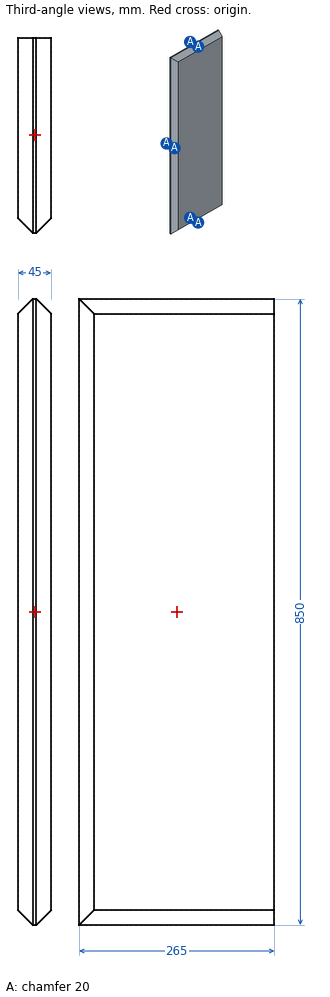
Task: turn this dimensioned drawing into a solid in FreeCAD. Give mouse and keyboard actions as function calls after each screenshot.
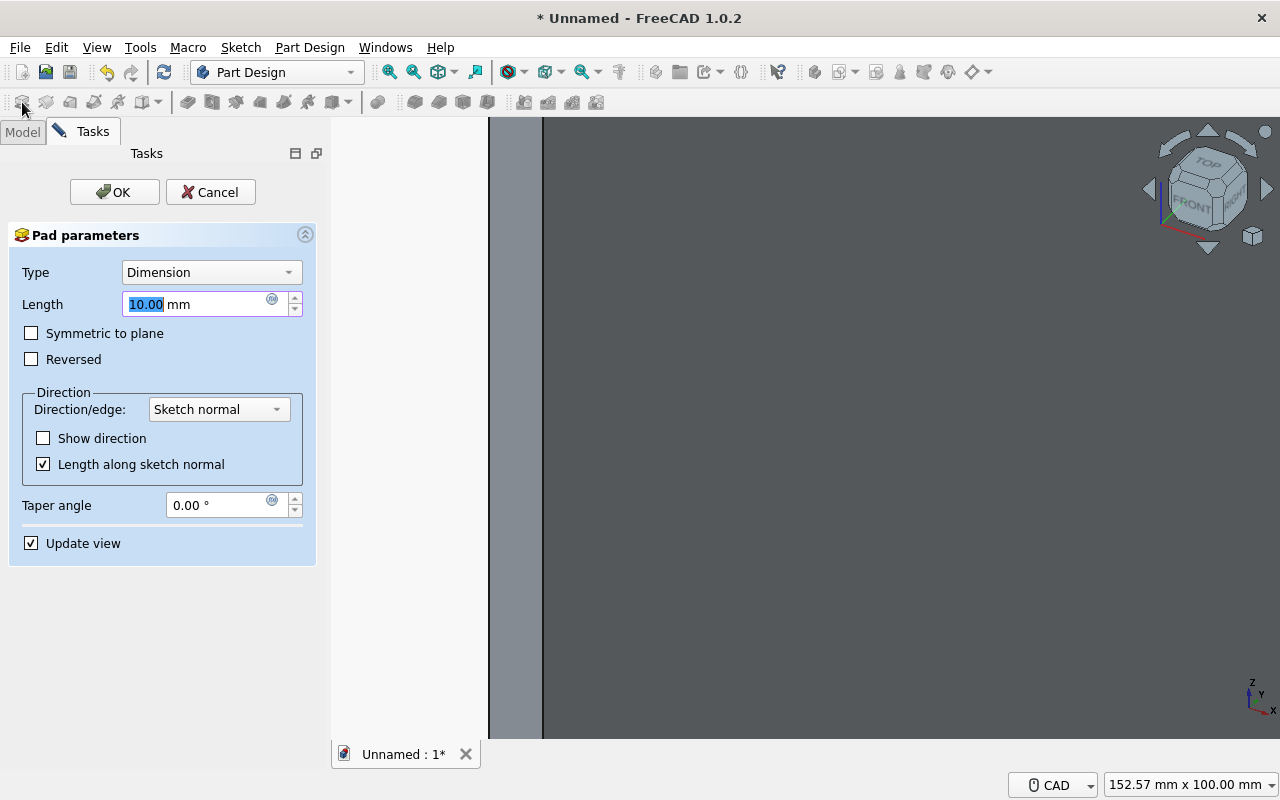
text(45)
key(Tab)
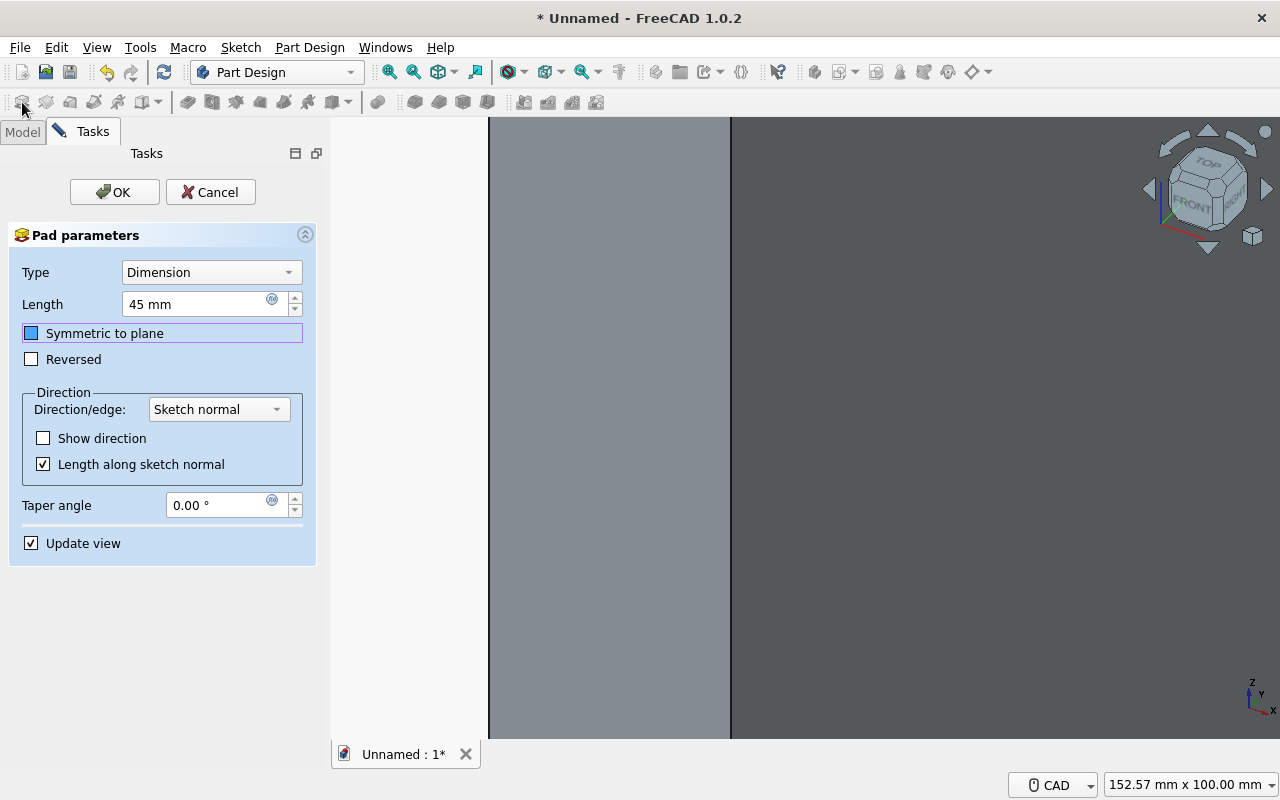
click(30, 333)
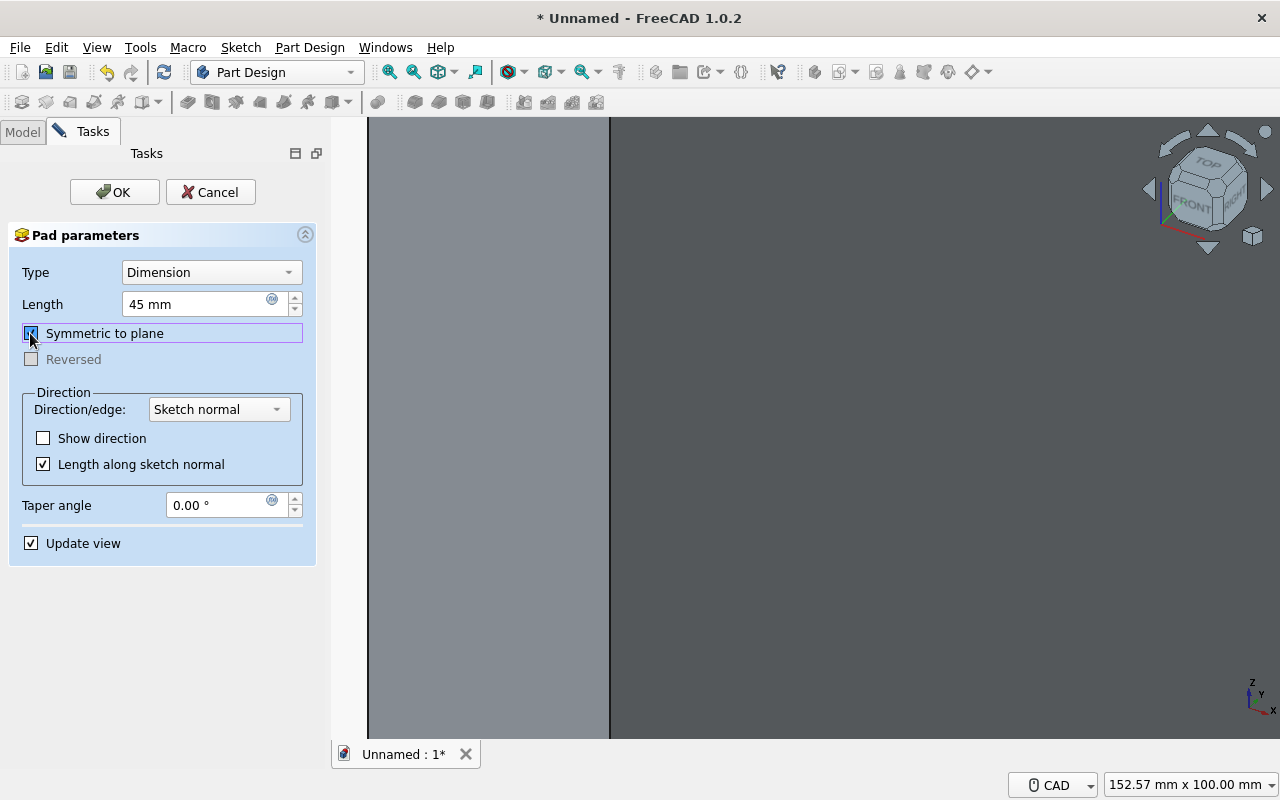
click(115, 192)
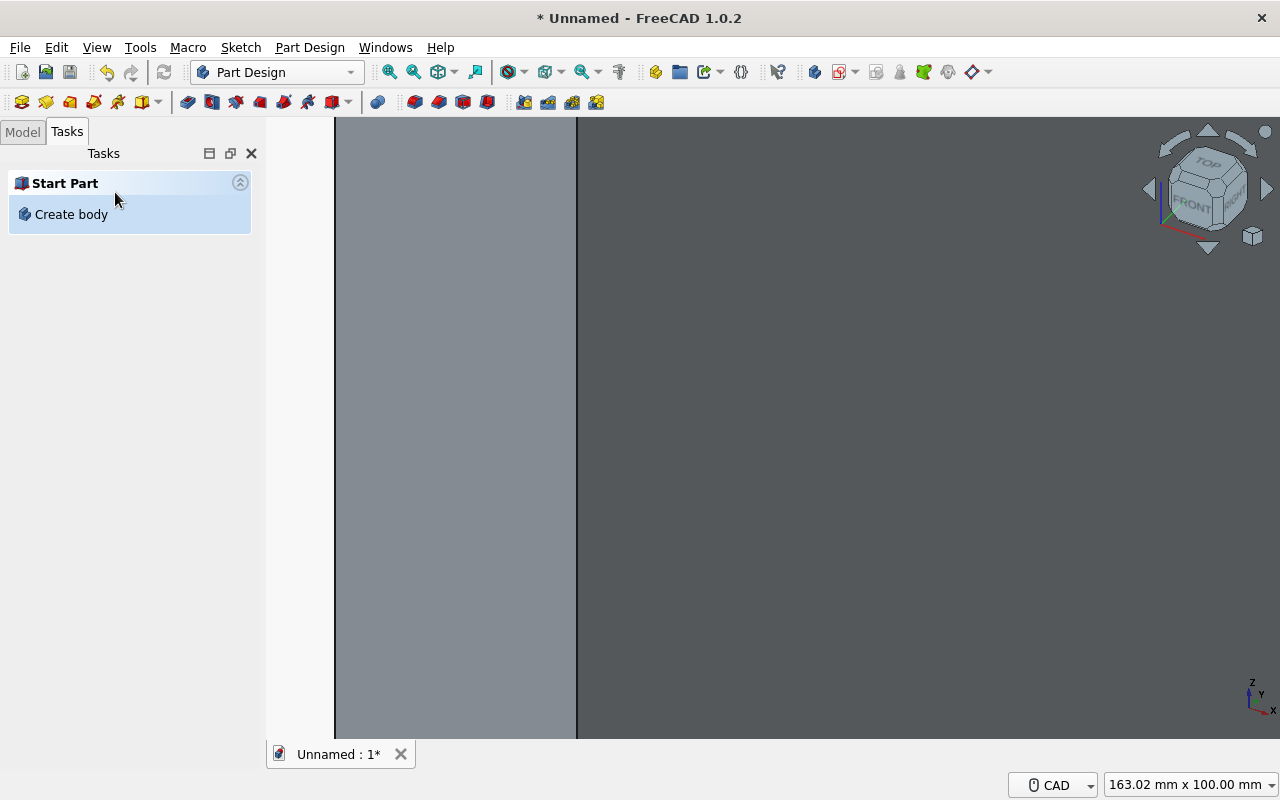
key(v)
key(f)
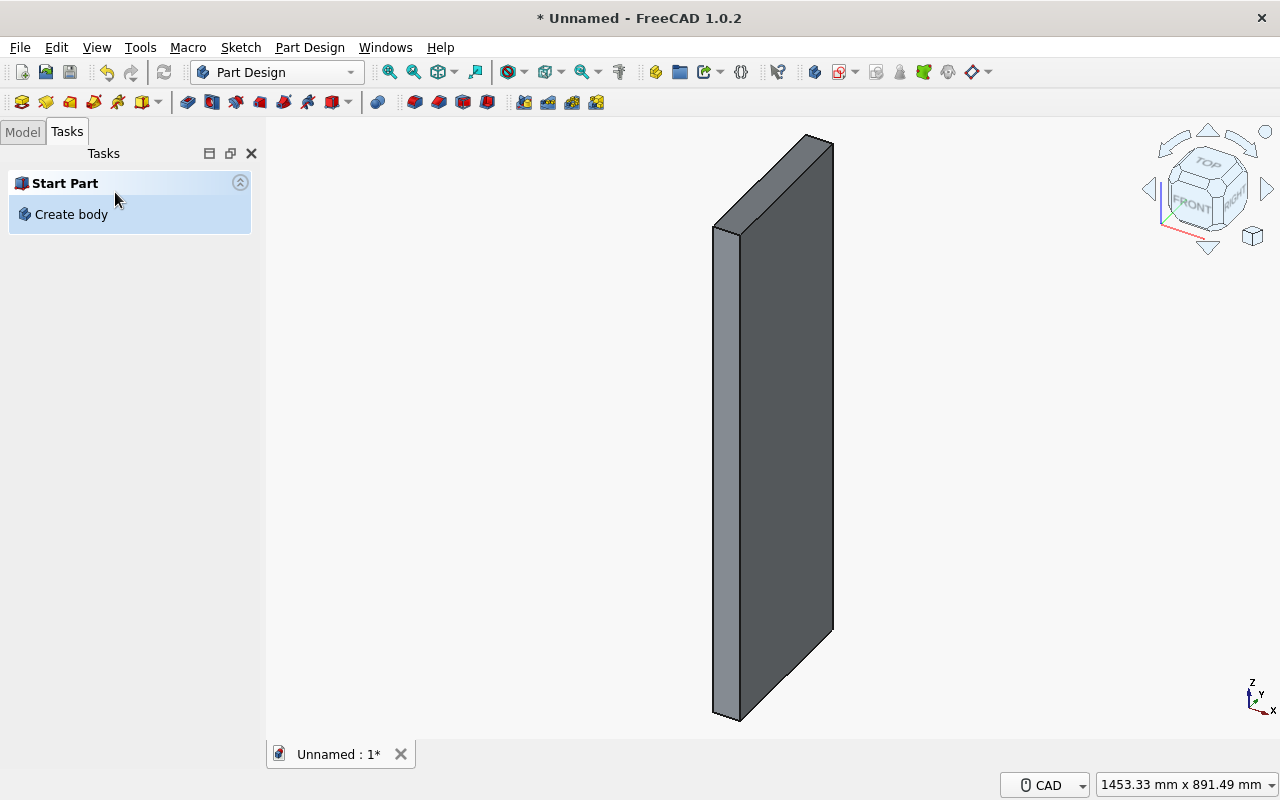
click(787, 189)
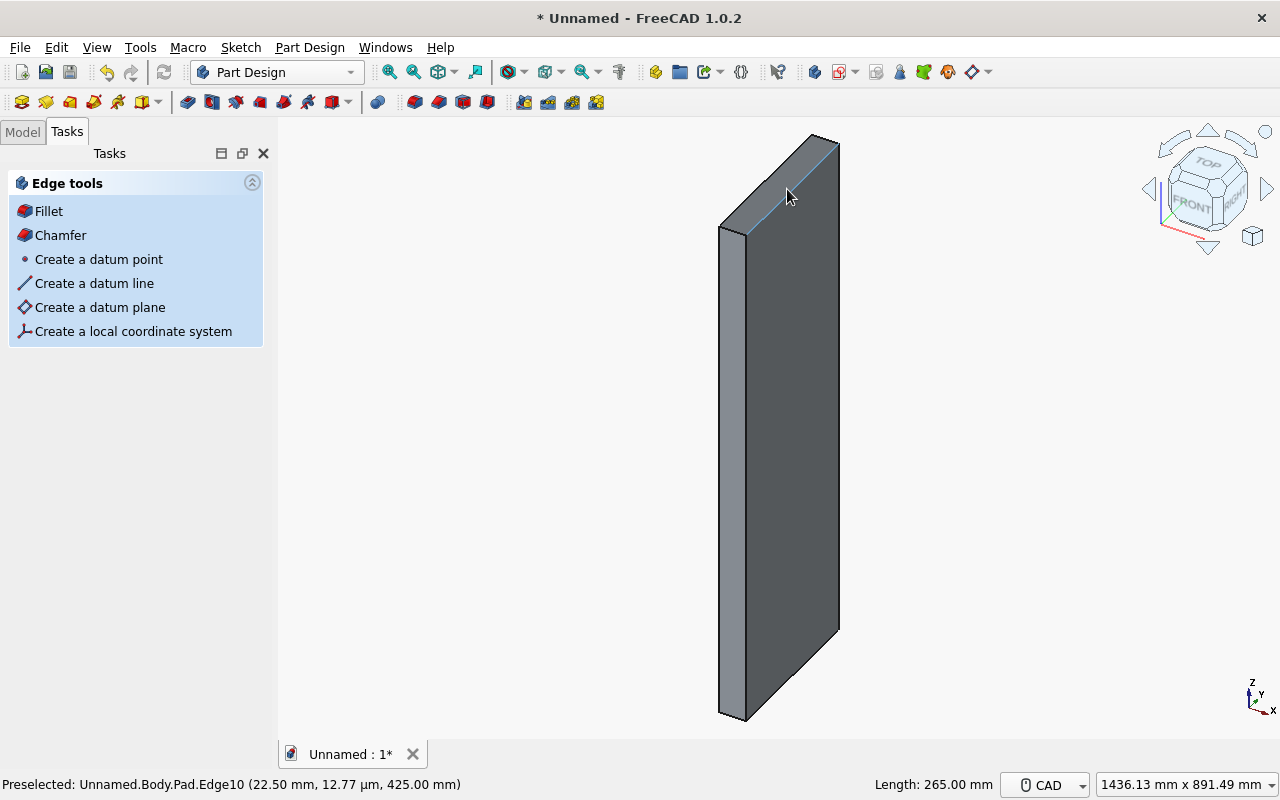
click(746, 477, ctrl)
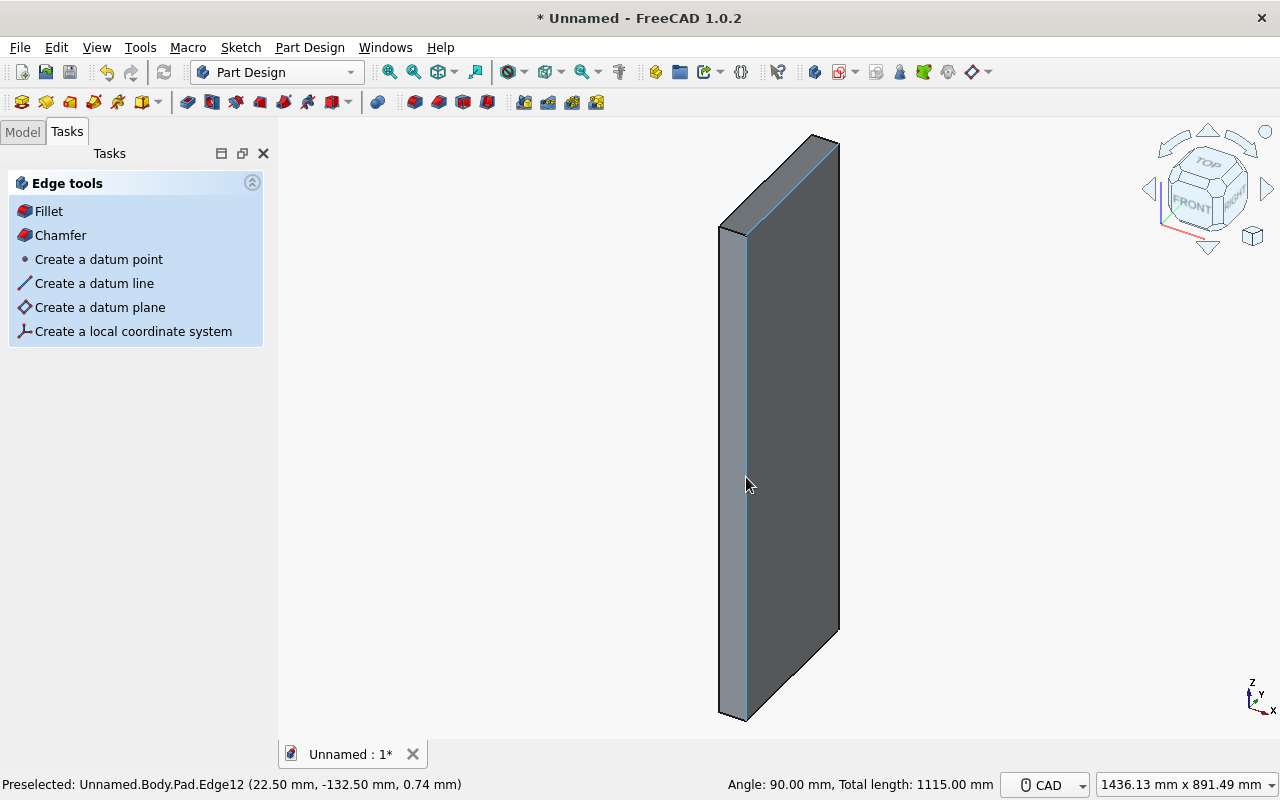
key(0)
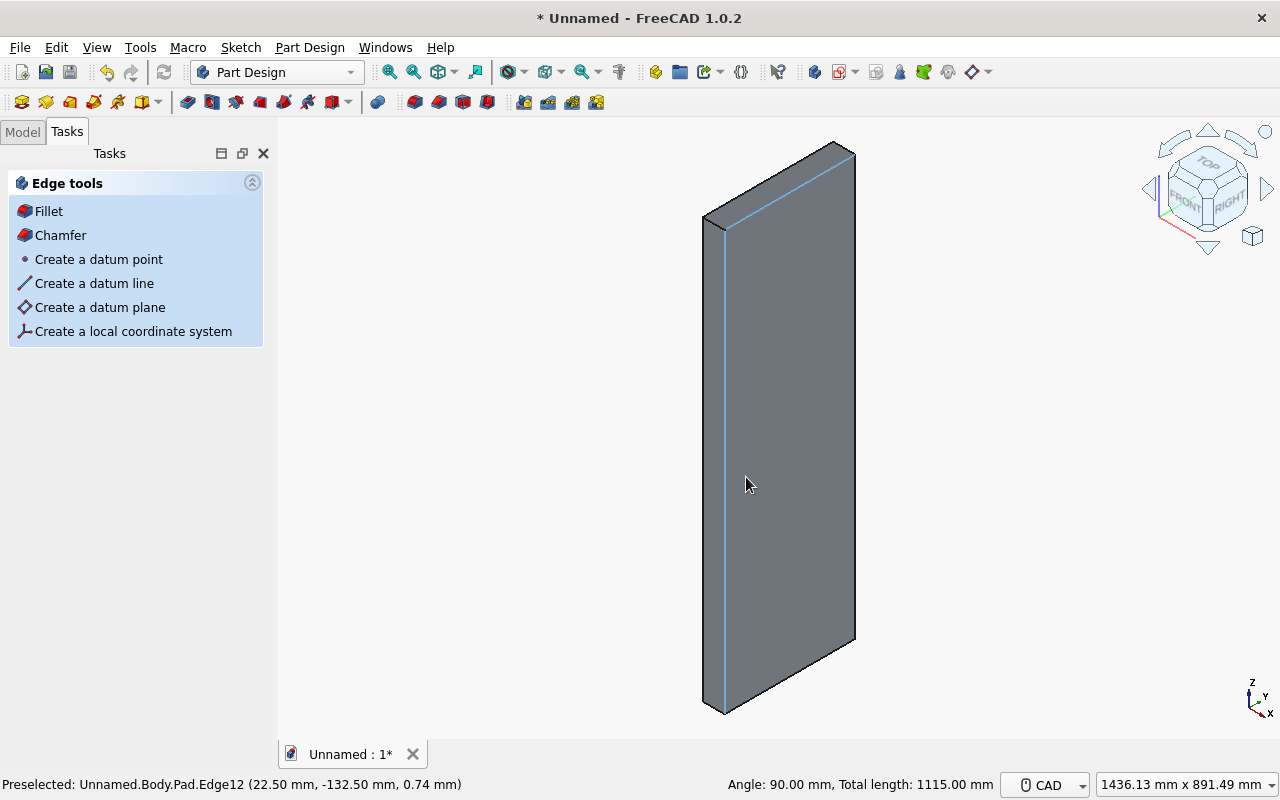
key(2)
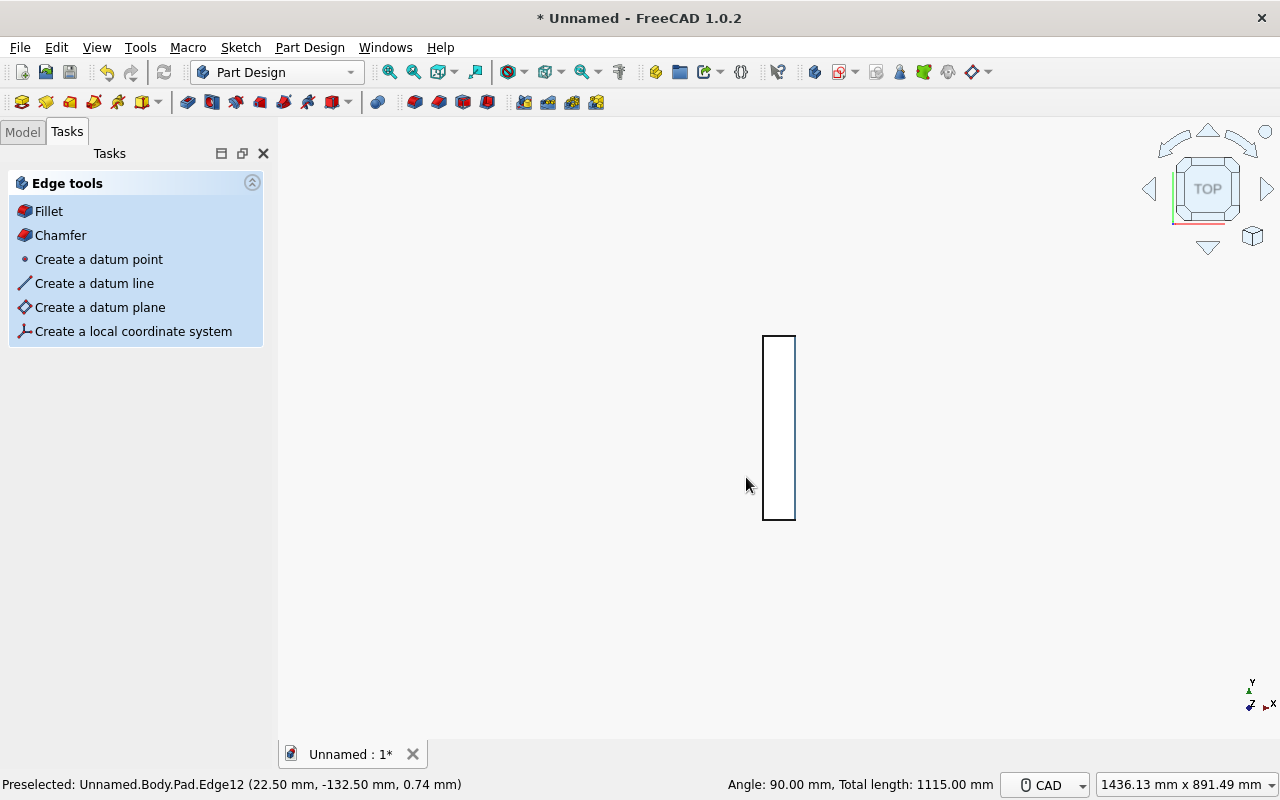
click(390, 72)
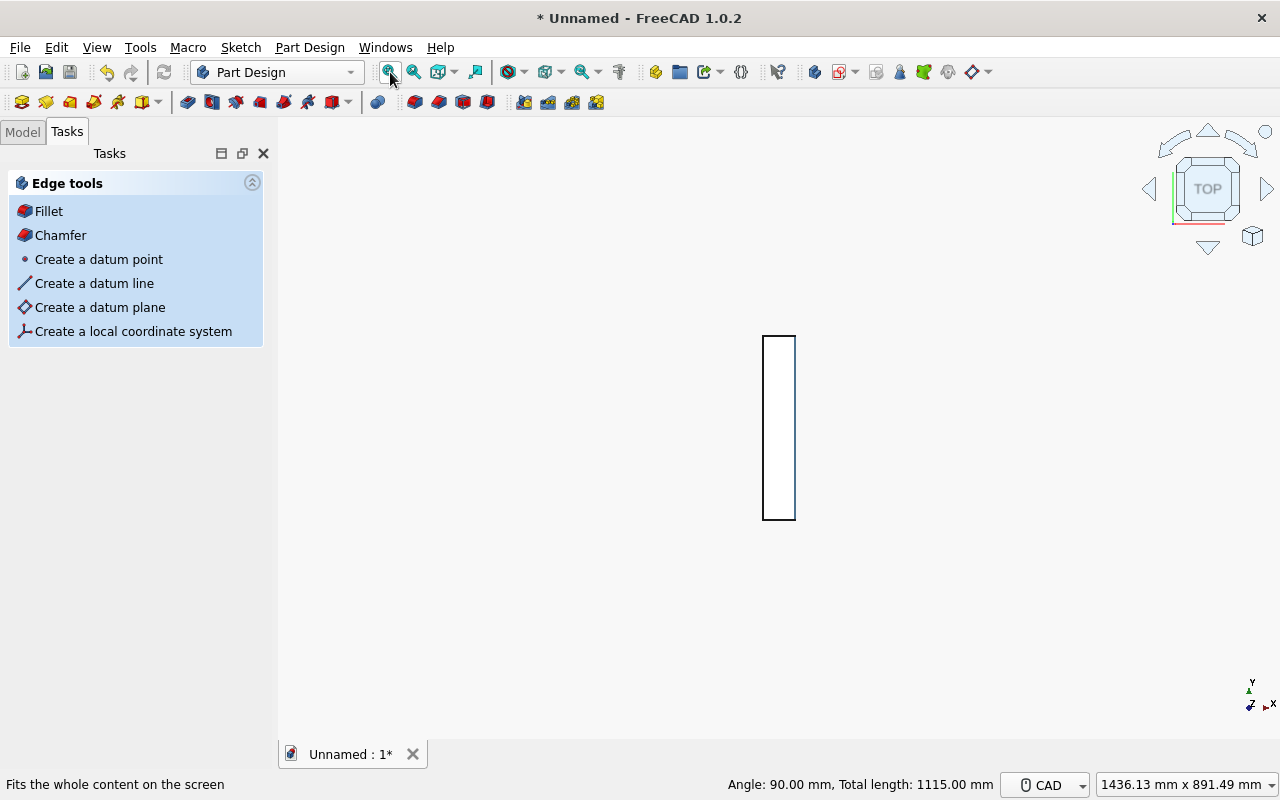
click(763, 427, ctrl)